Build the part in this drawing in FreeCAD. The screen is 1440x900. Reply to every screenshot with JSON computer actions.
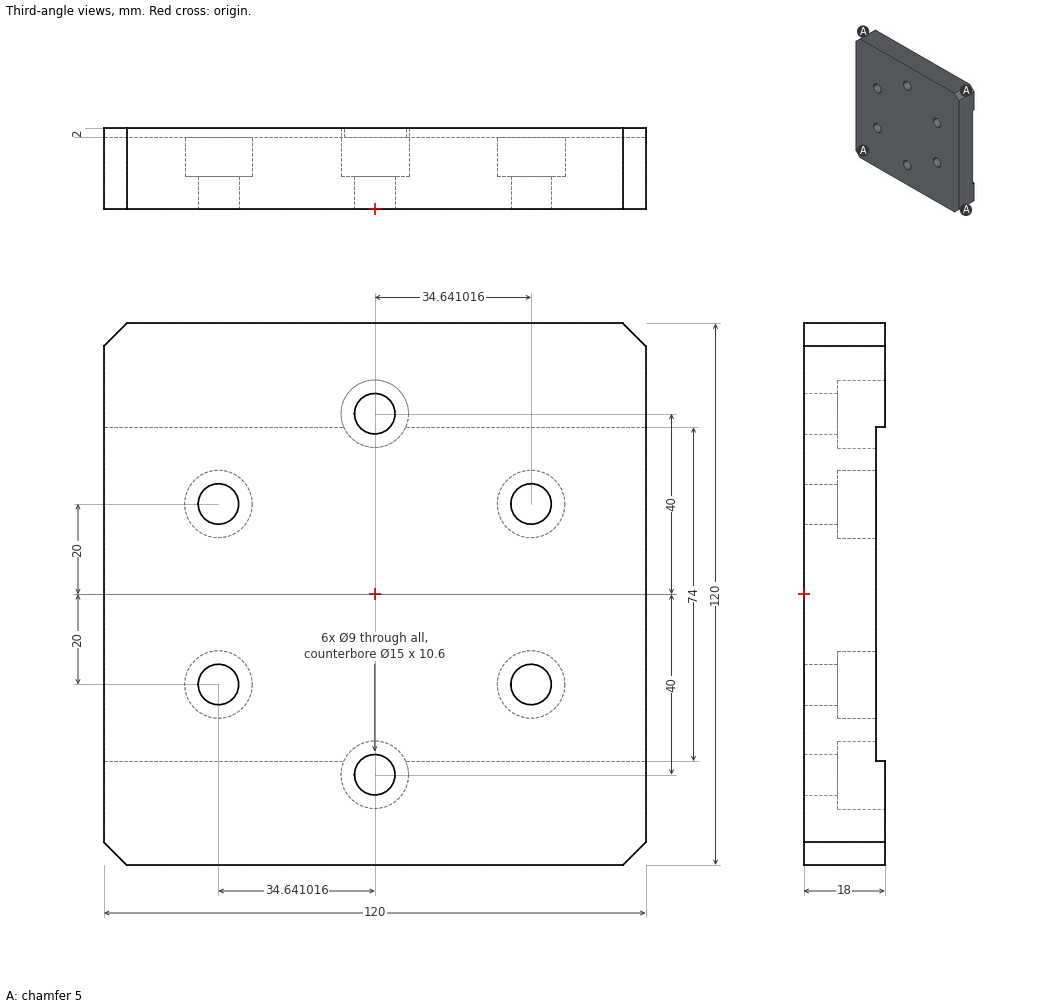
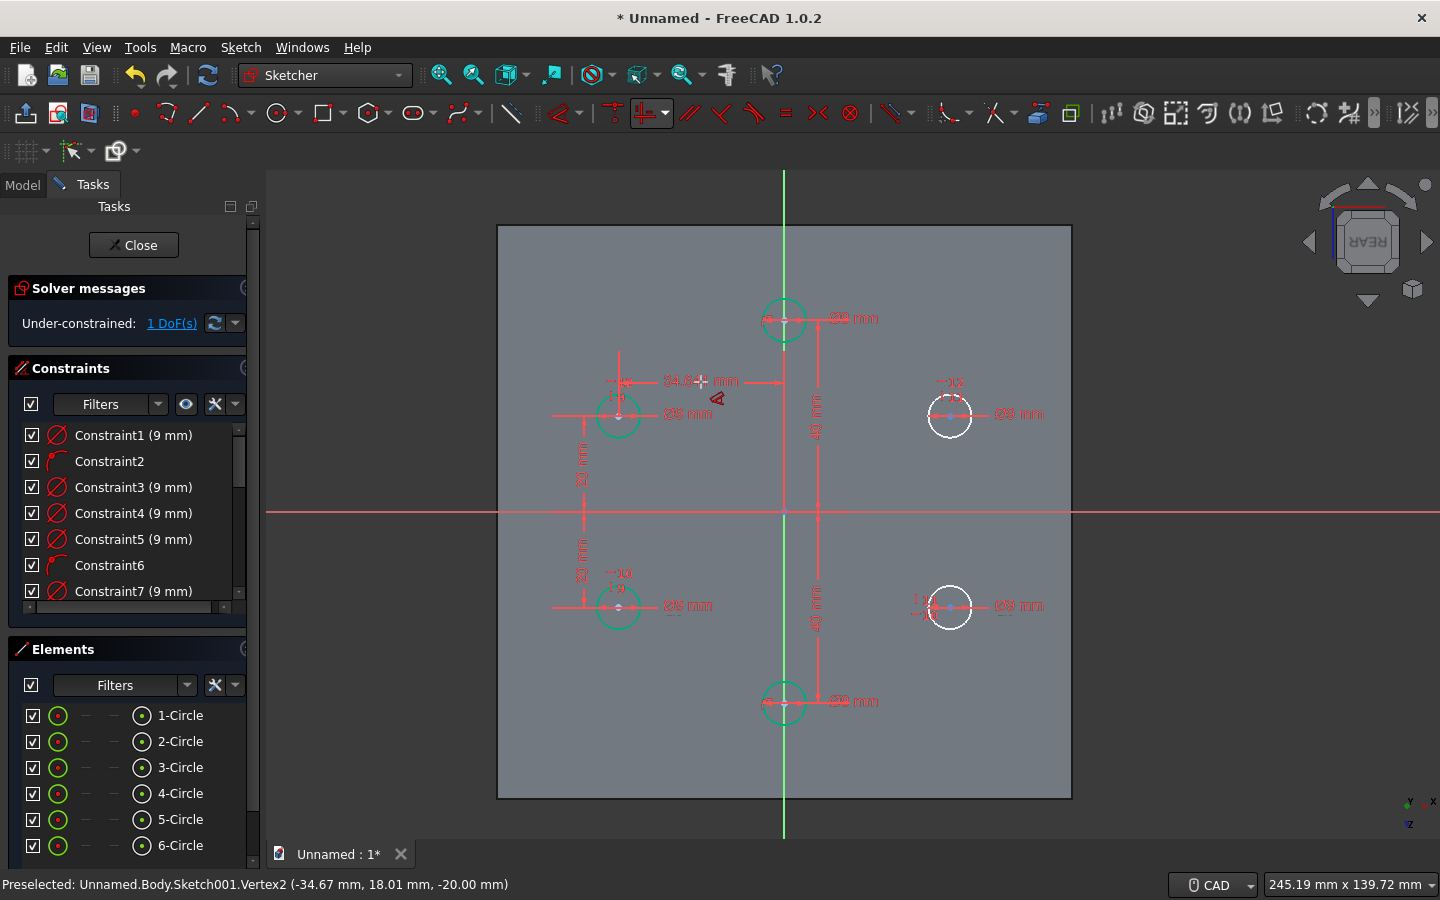
{"action": "left_click", "coordinate": [950, 608]}
{"action": "left_click", "coordinate": [867, 642]}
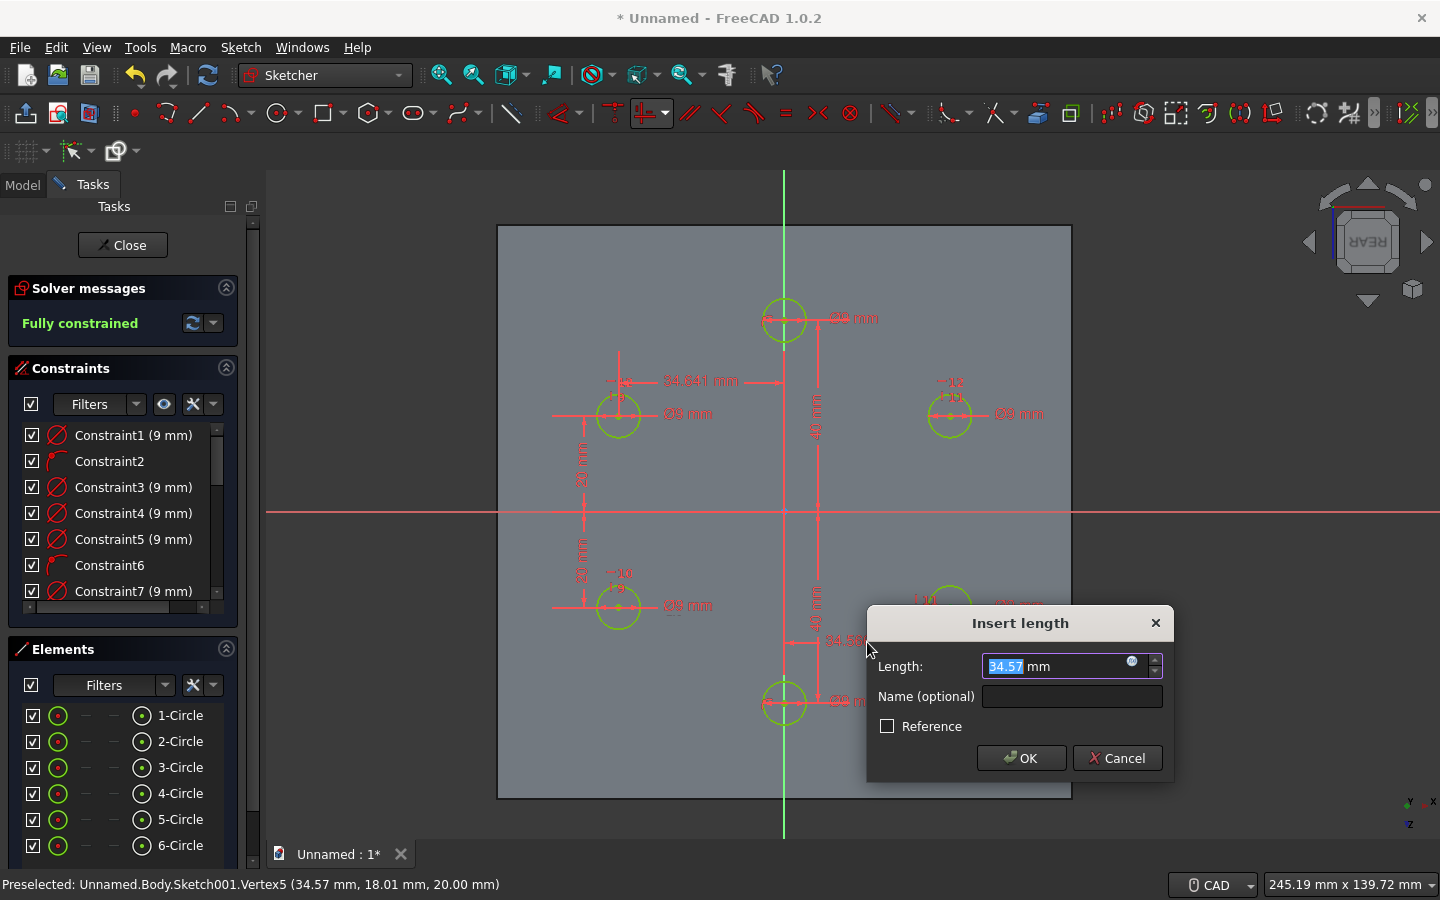
{"action": "type", "text": "34.641016"}
{"action": "key", "text": "Return"}
{"action": "key", "text": "Escape"}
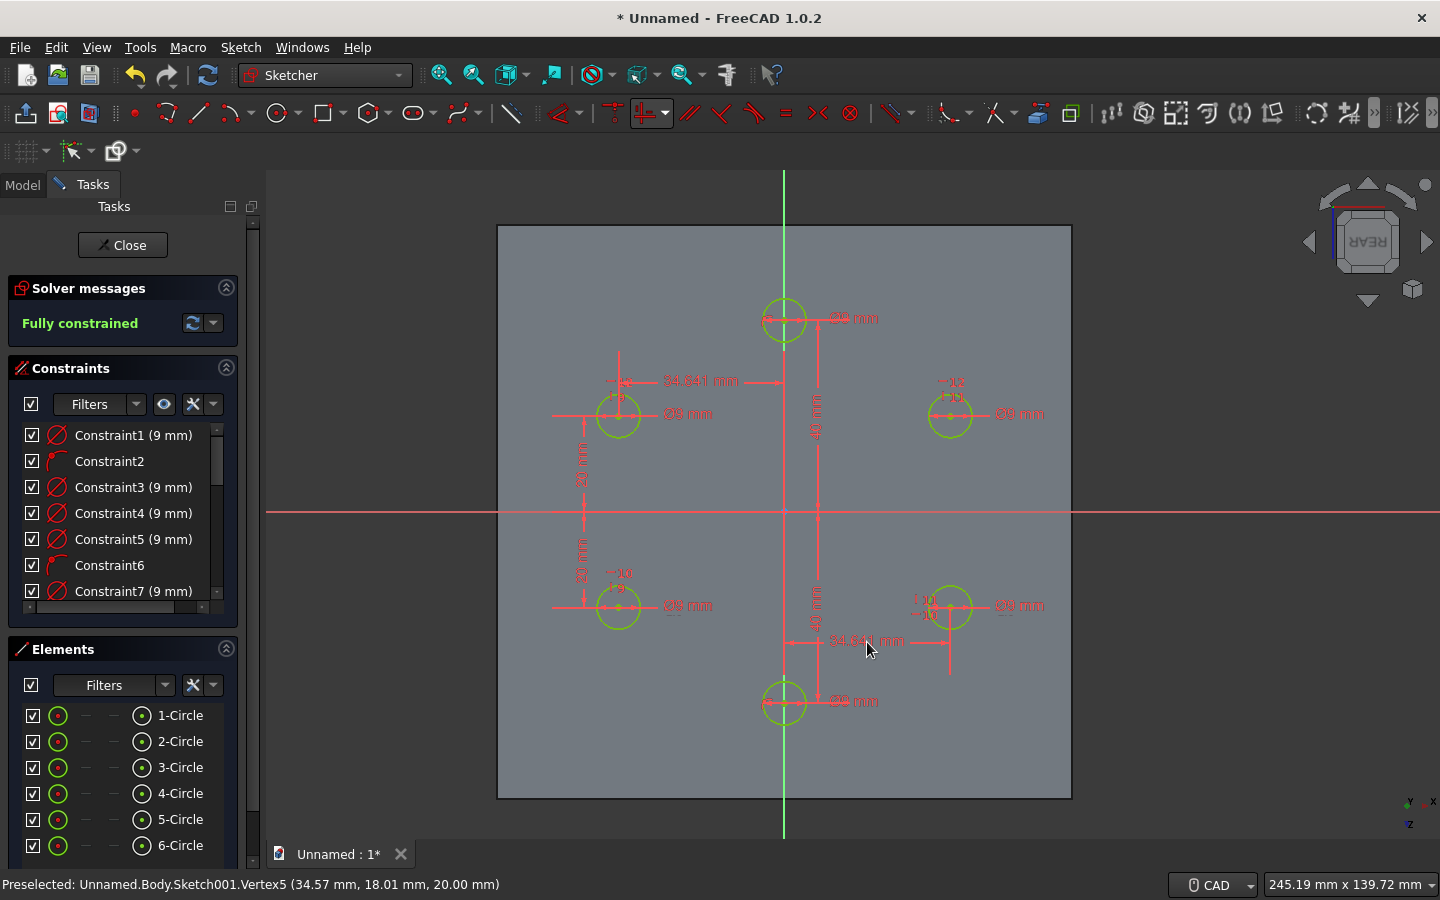
{"action": "left_click", "coordinate": [123, 245]}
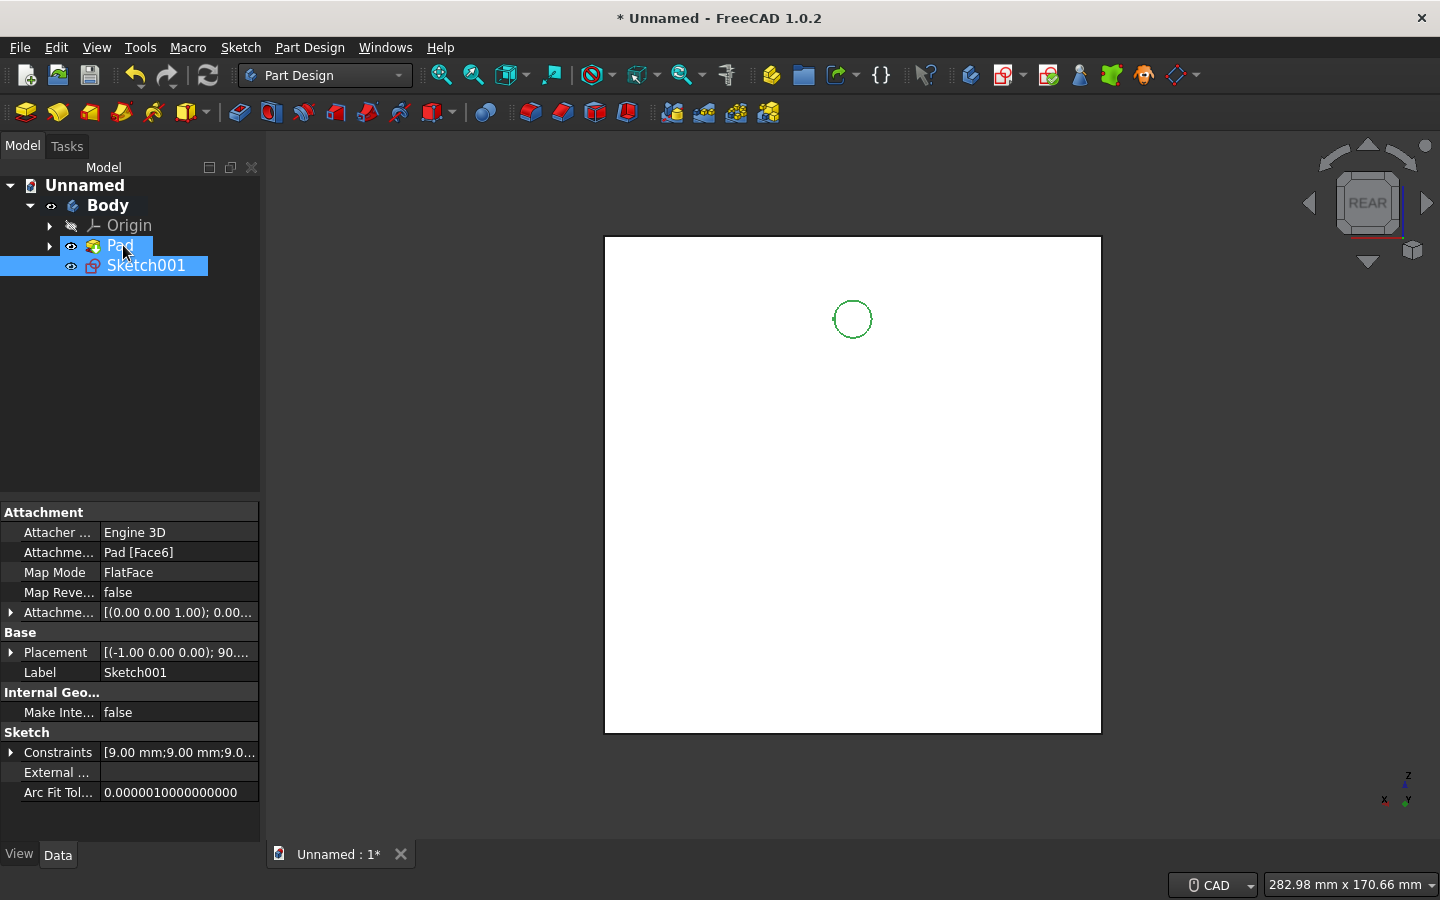
{"action": "left_click", "coordinate": [272, 112]}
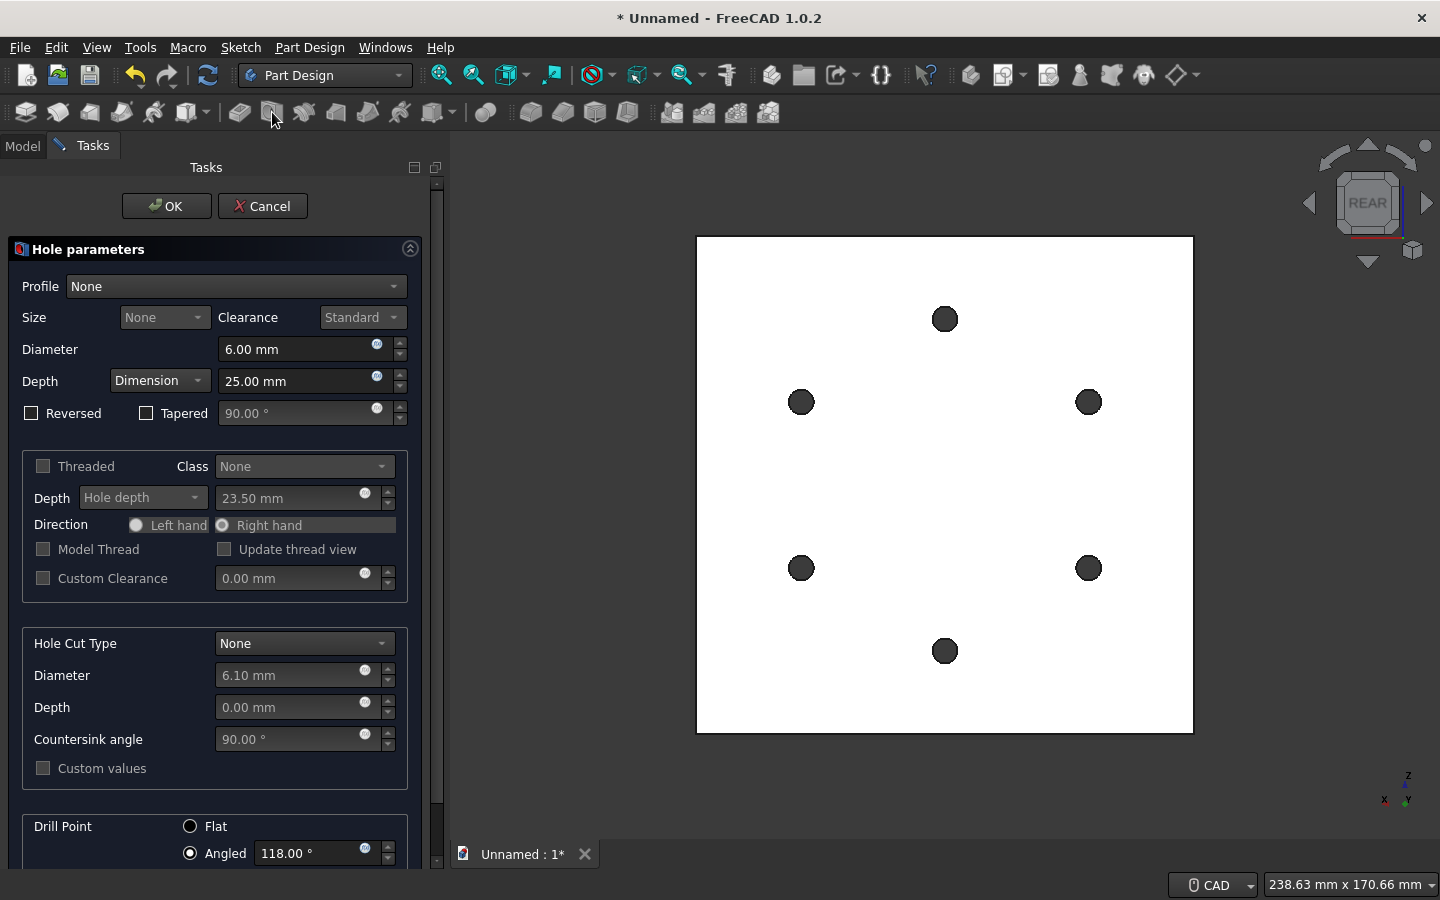
{"action": "triple_click", "coordinate": [305, 349]}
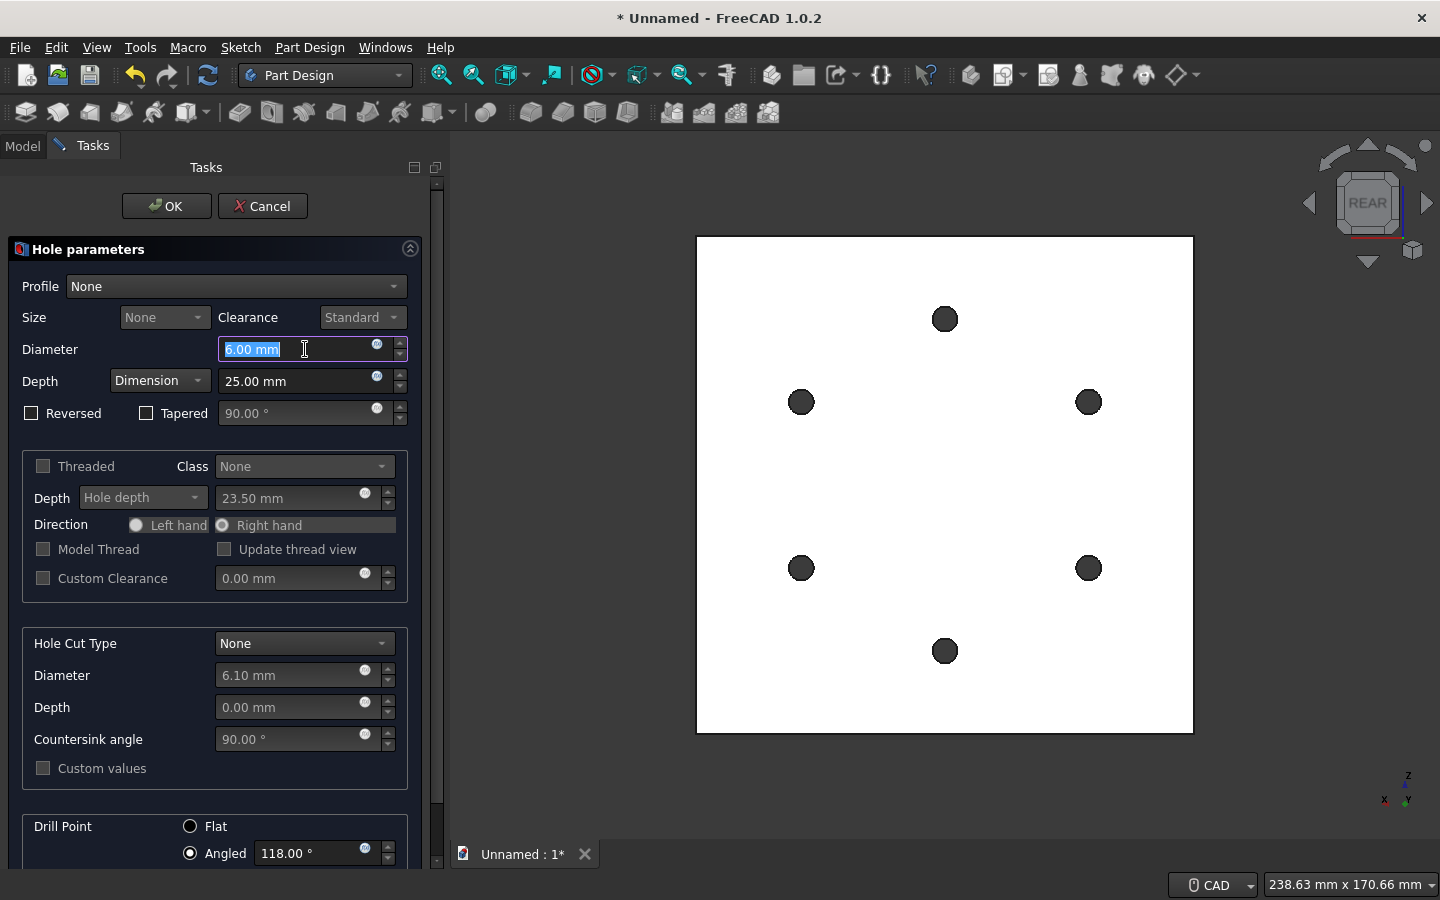
{"action": "type", "text": "9"}
{"action": "key", "text": "Tab"}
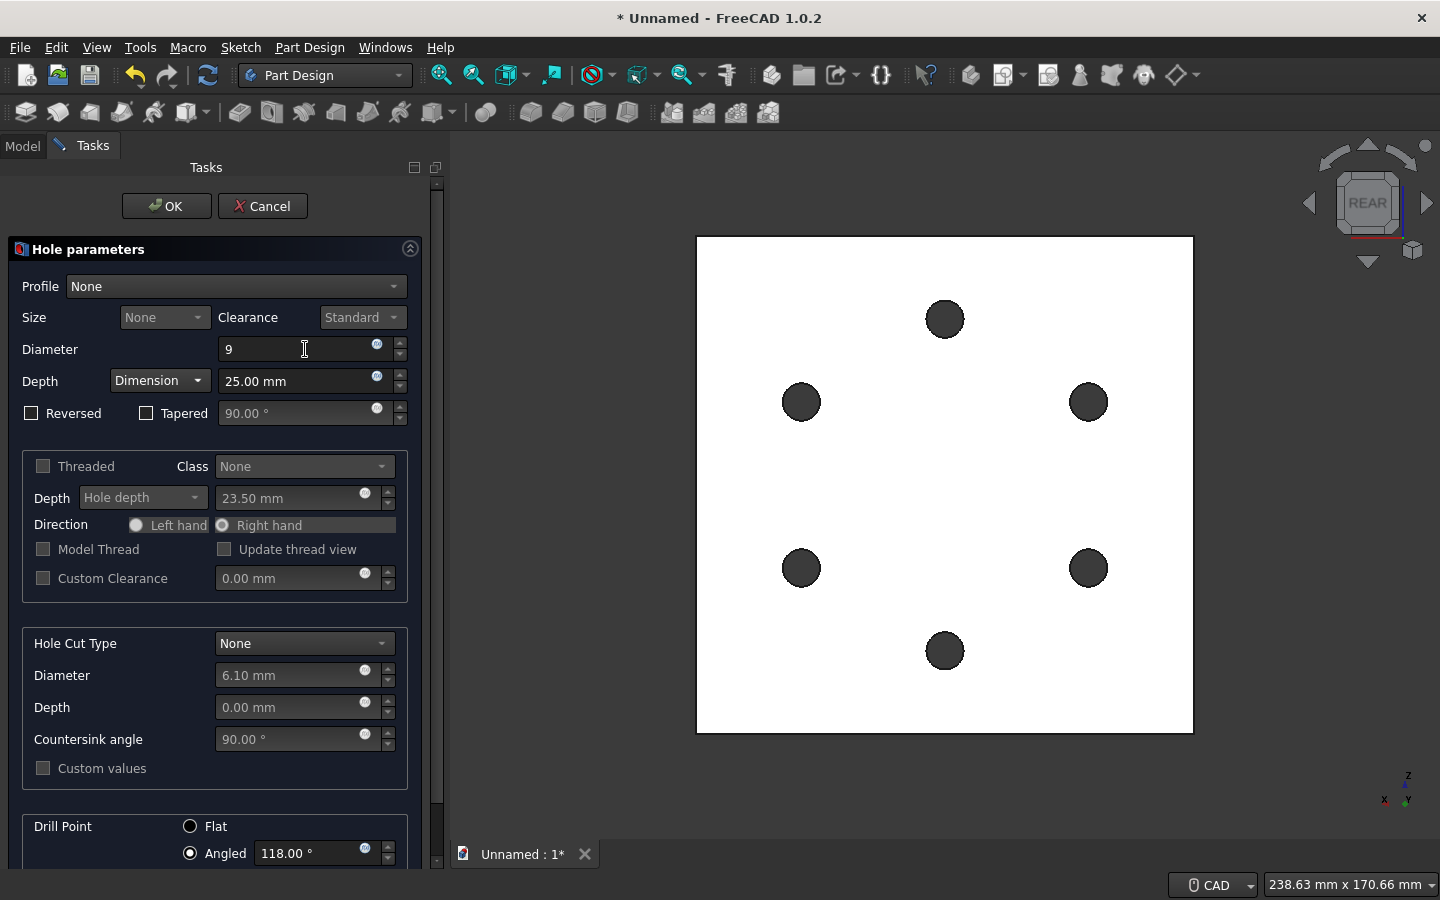
{"action": "left_click", "coordinate": [161, 380]}